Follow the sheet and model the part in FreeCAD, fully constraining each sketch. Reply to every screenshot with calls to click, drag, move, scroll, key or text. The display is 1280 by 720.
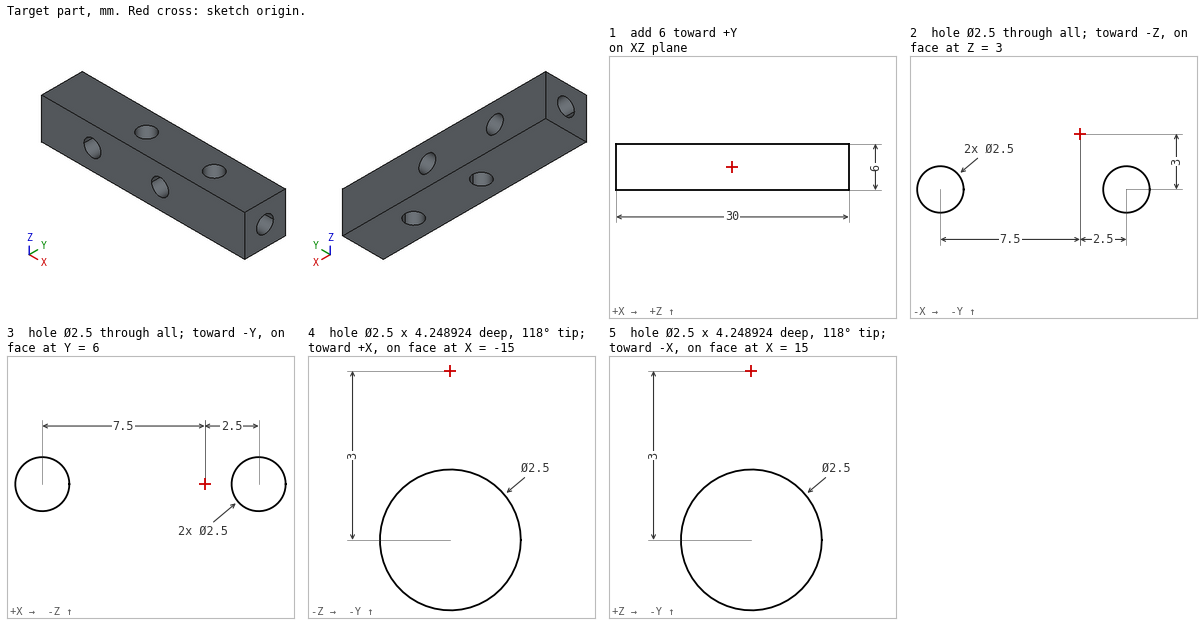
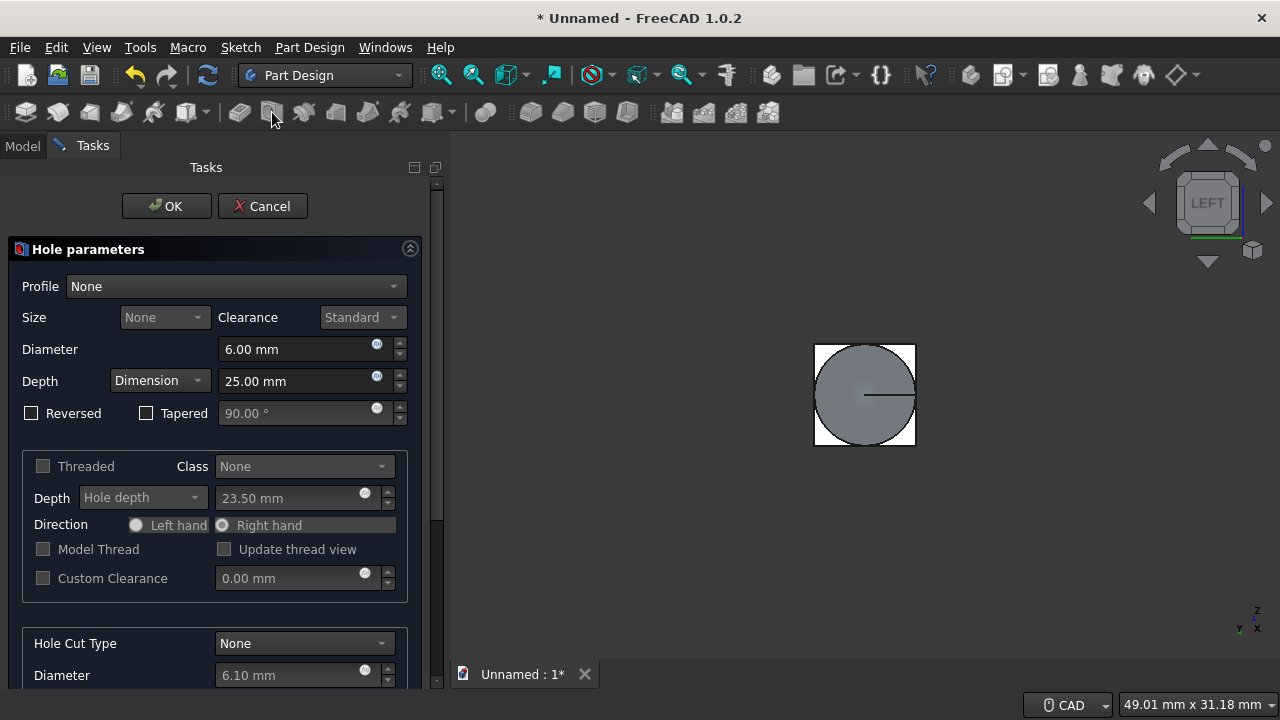
triple_click(305, 349)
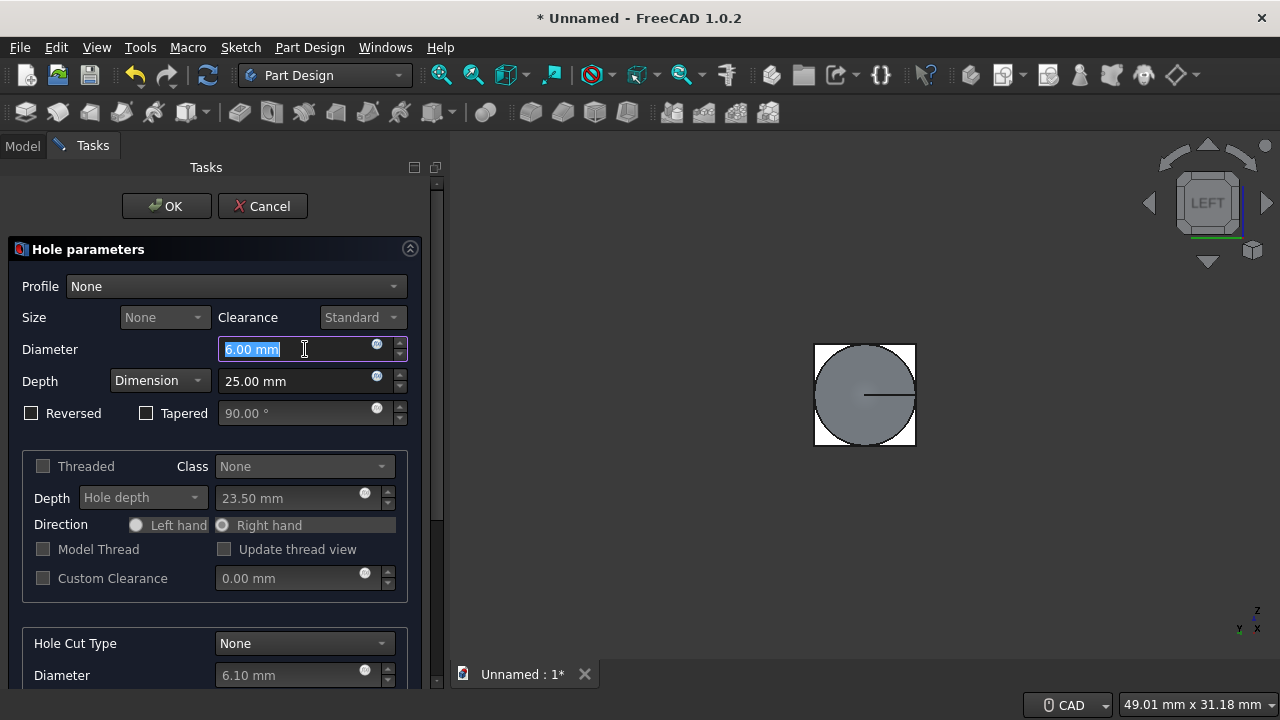
text(2.5)
key(Tab)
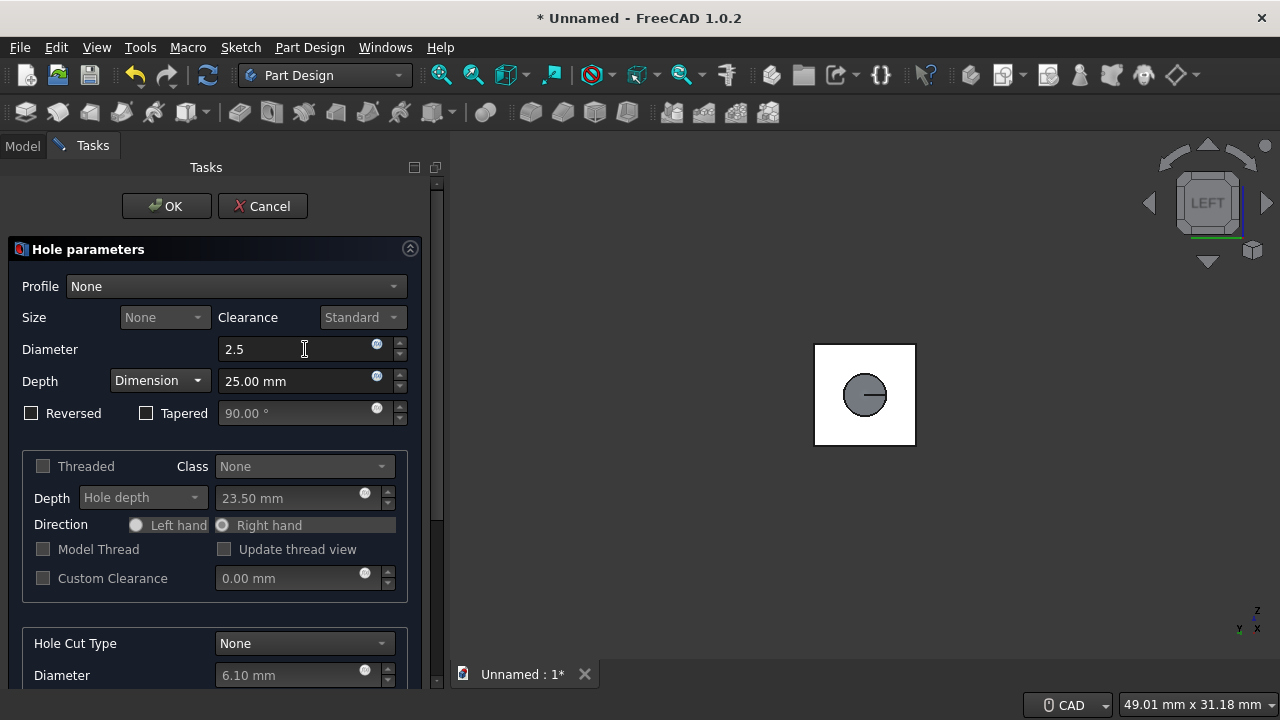
triple_click(305, 381)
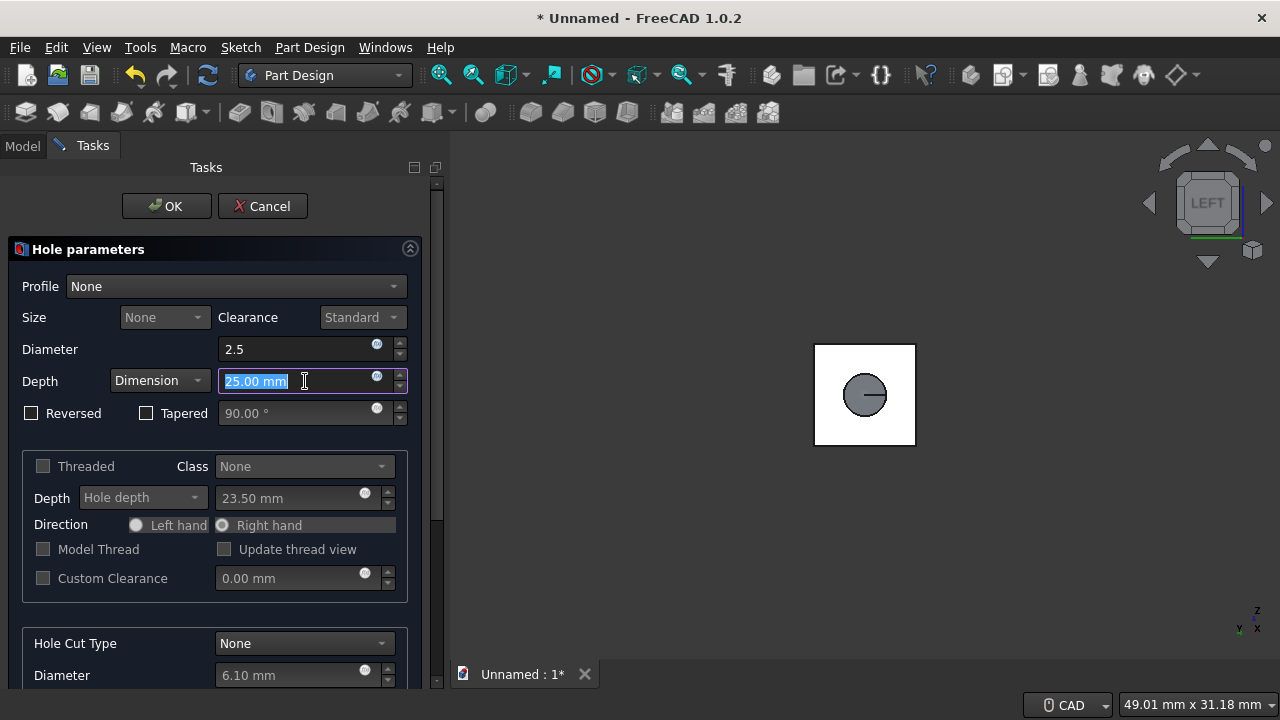
text(4.248924)
key(Tab)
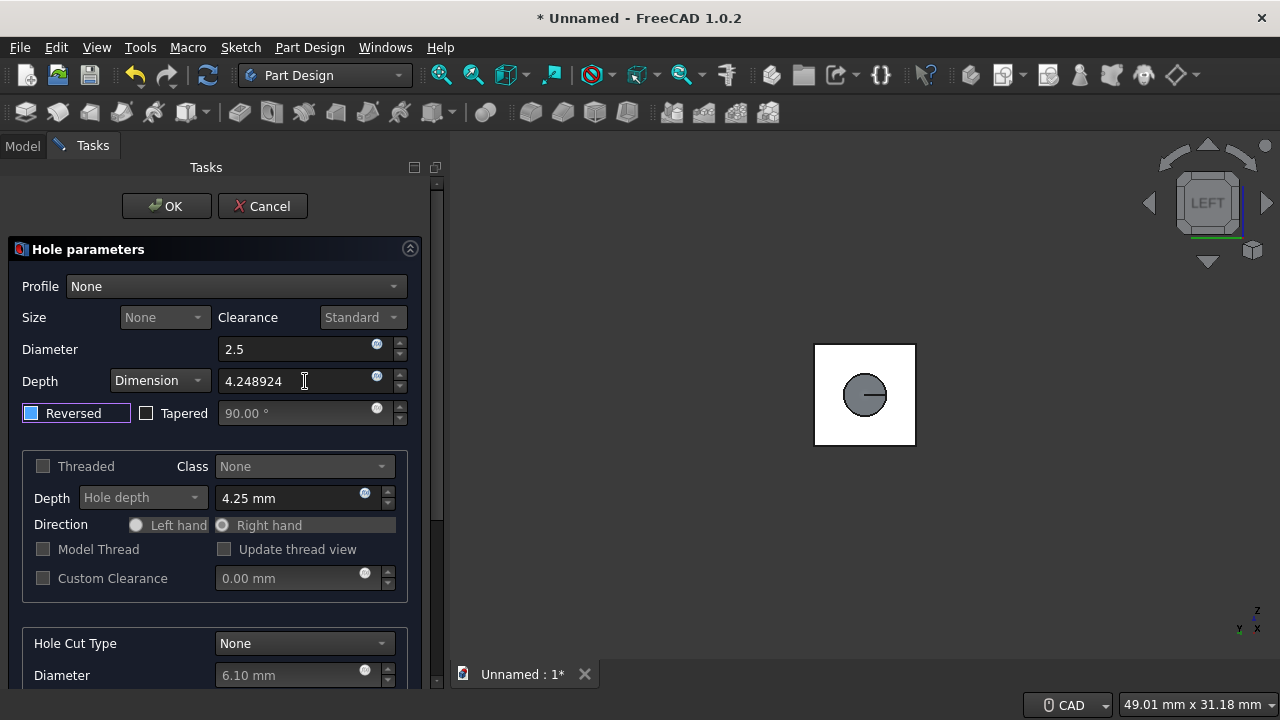
click(167, 206)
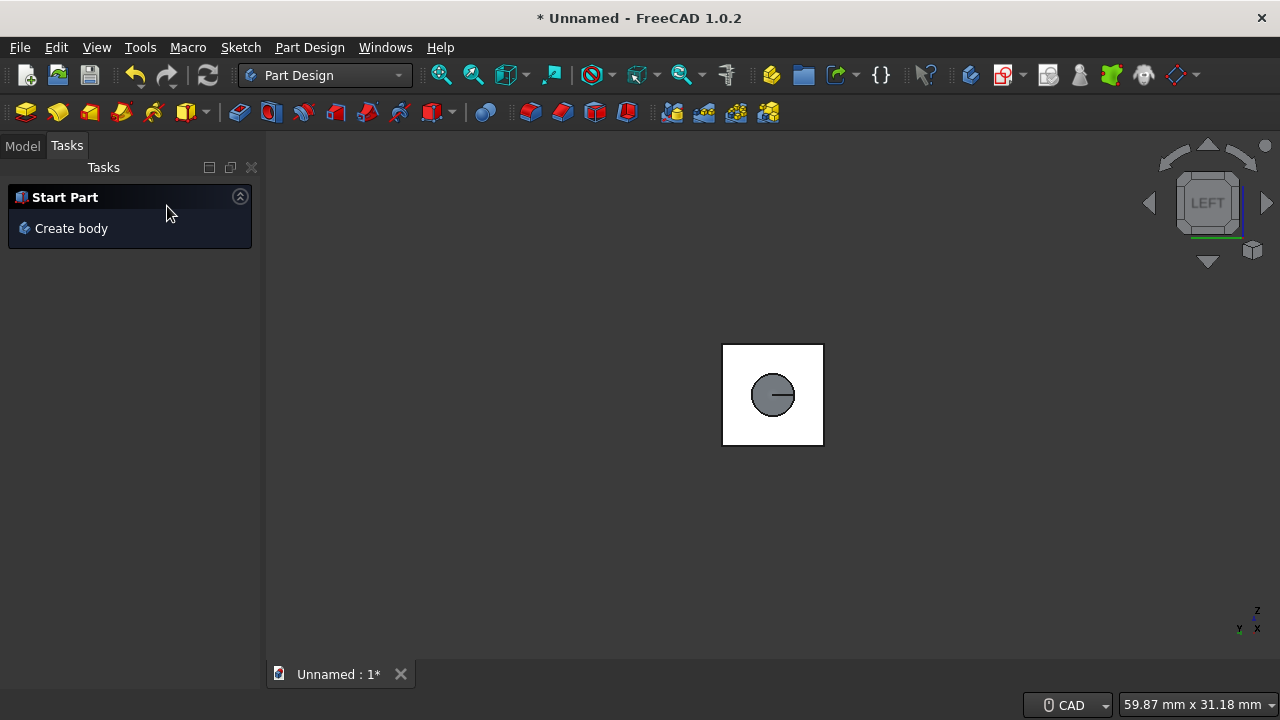
click(442, 76)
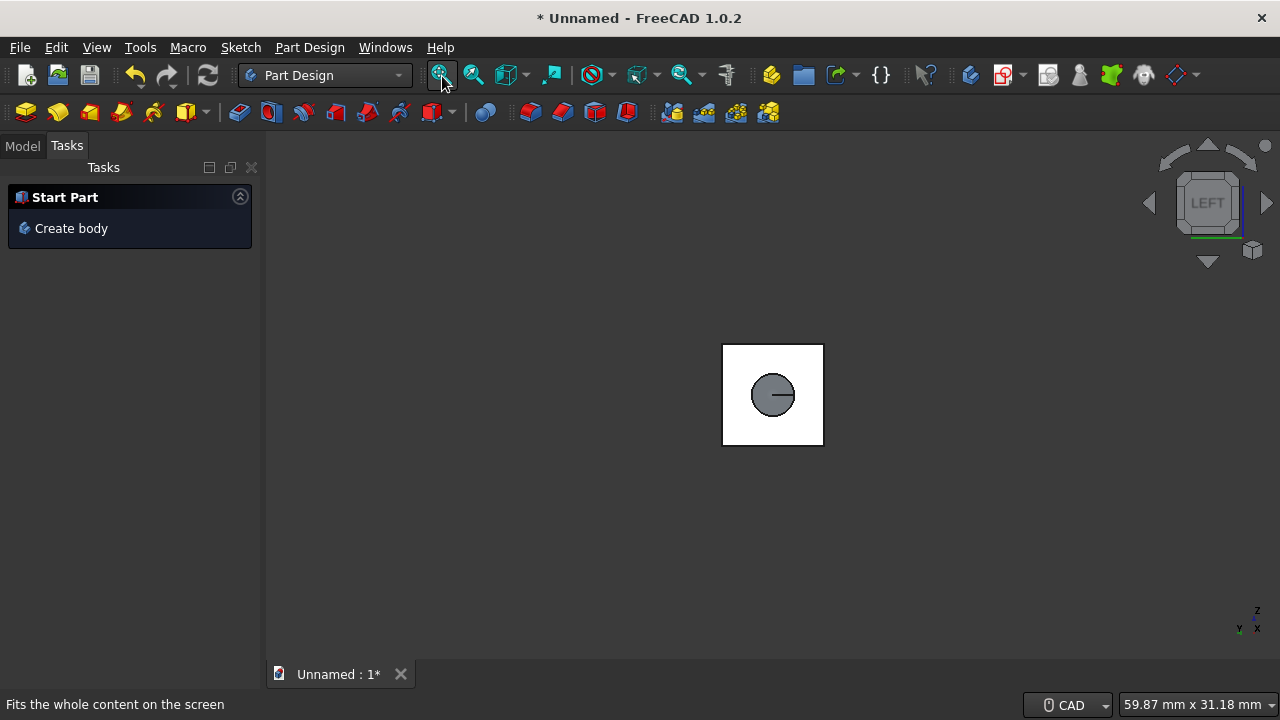
key(0)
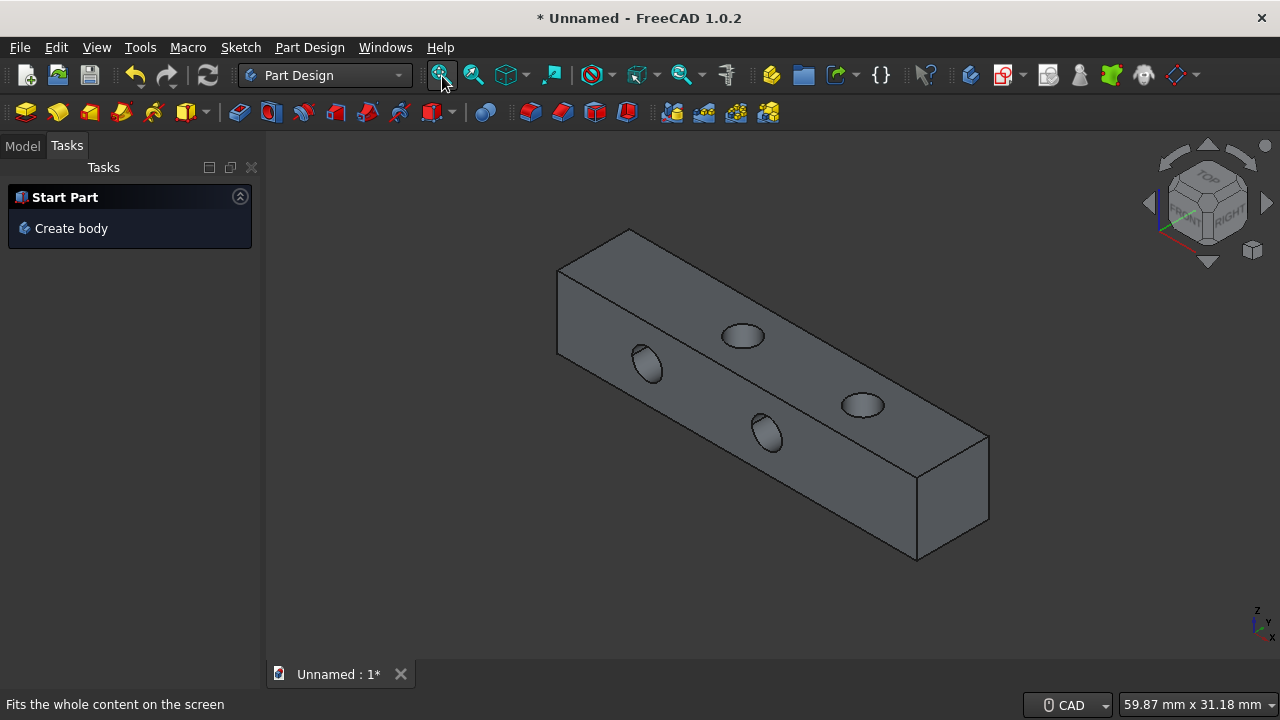
click(953, 498)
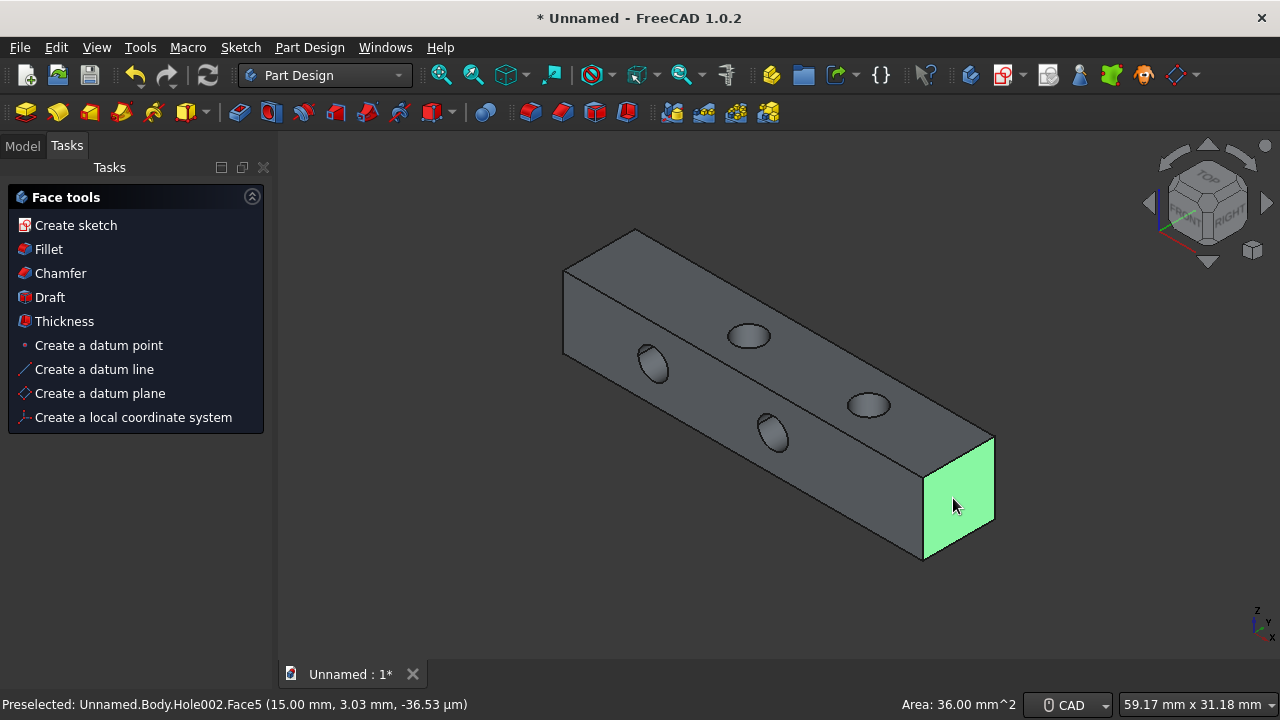
click(1004, 76)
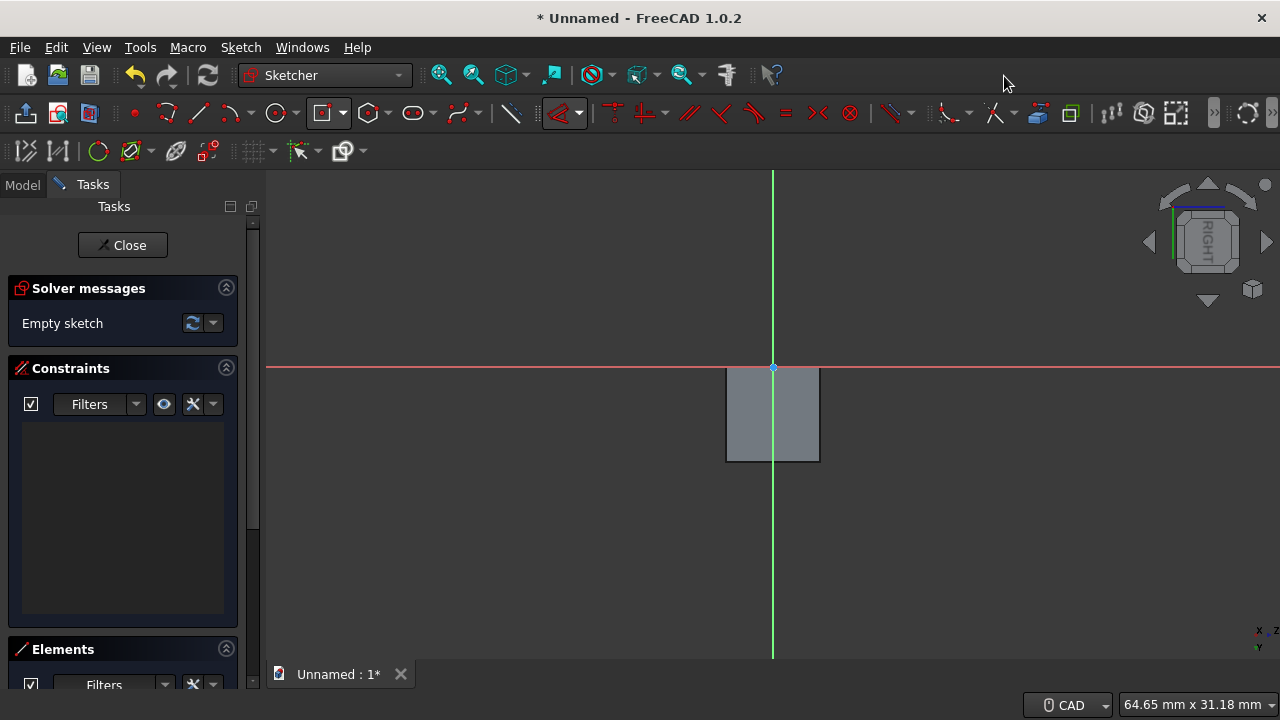
scroll(790, 397, up, 8)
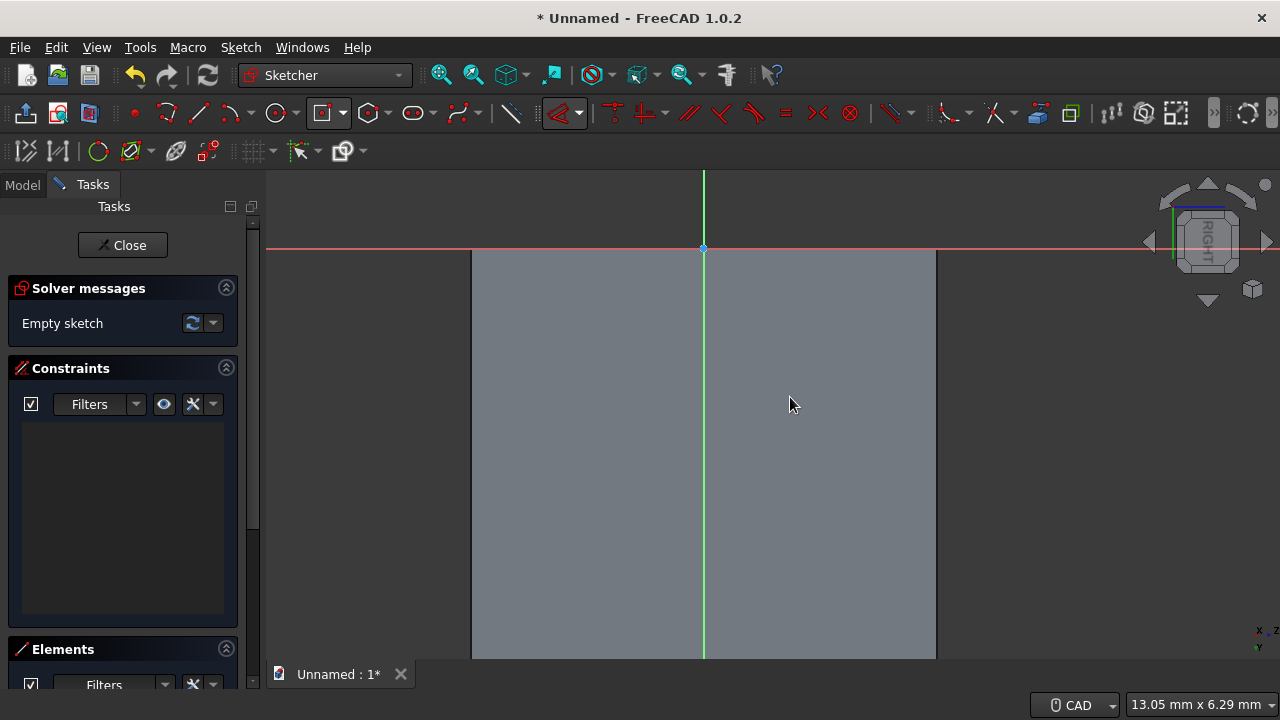
key(g)
key(c)